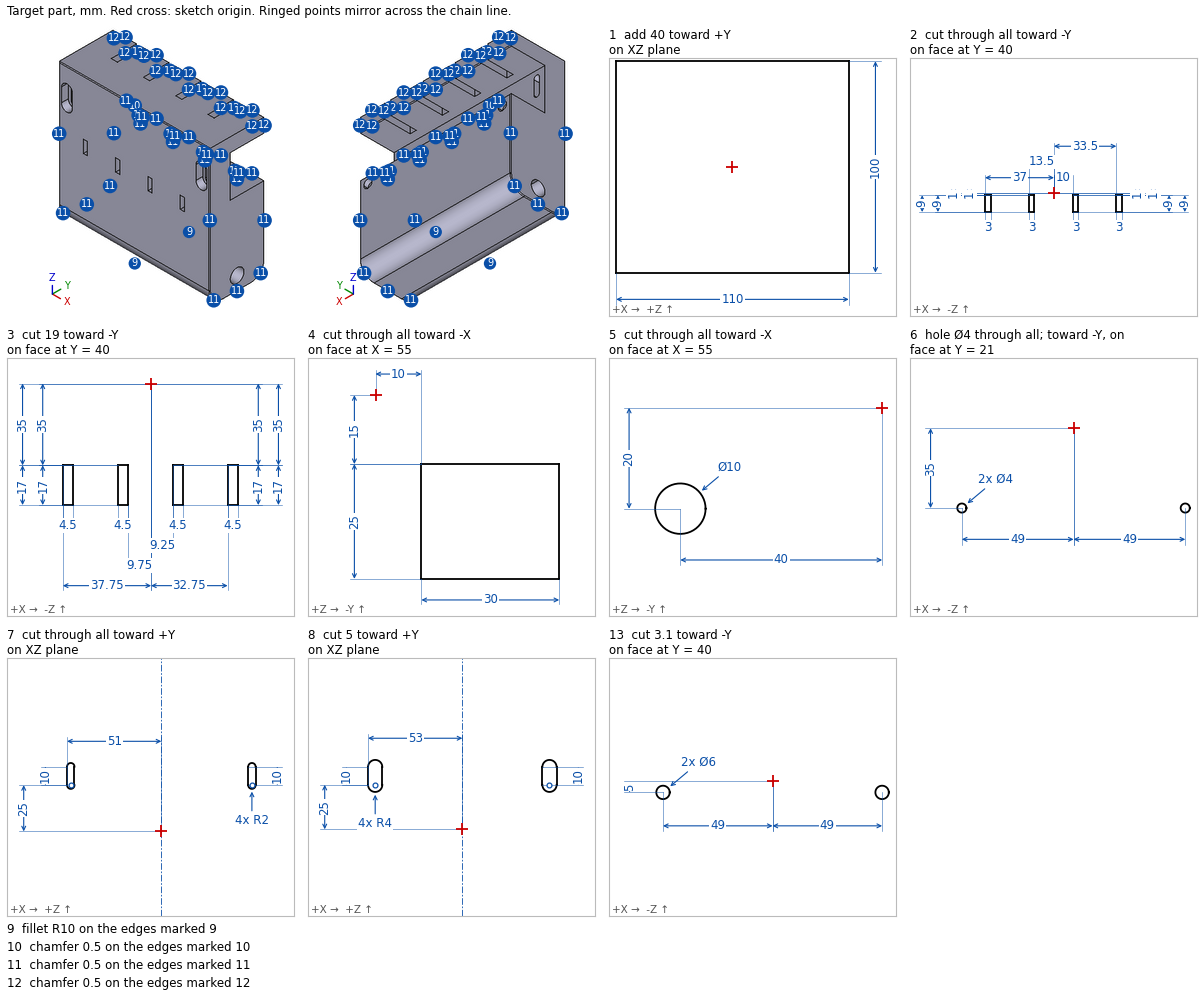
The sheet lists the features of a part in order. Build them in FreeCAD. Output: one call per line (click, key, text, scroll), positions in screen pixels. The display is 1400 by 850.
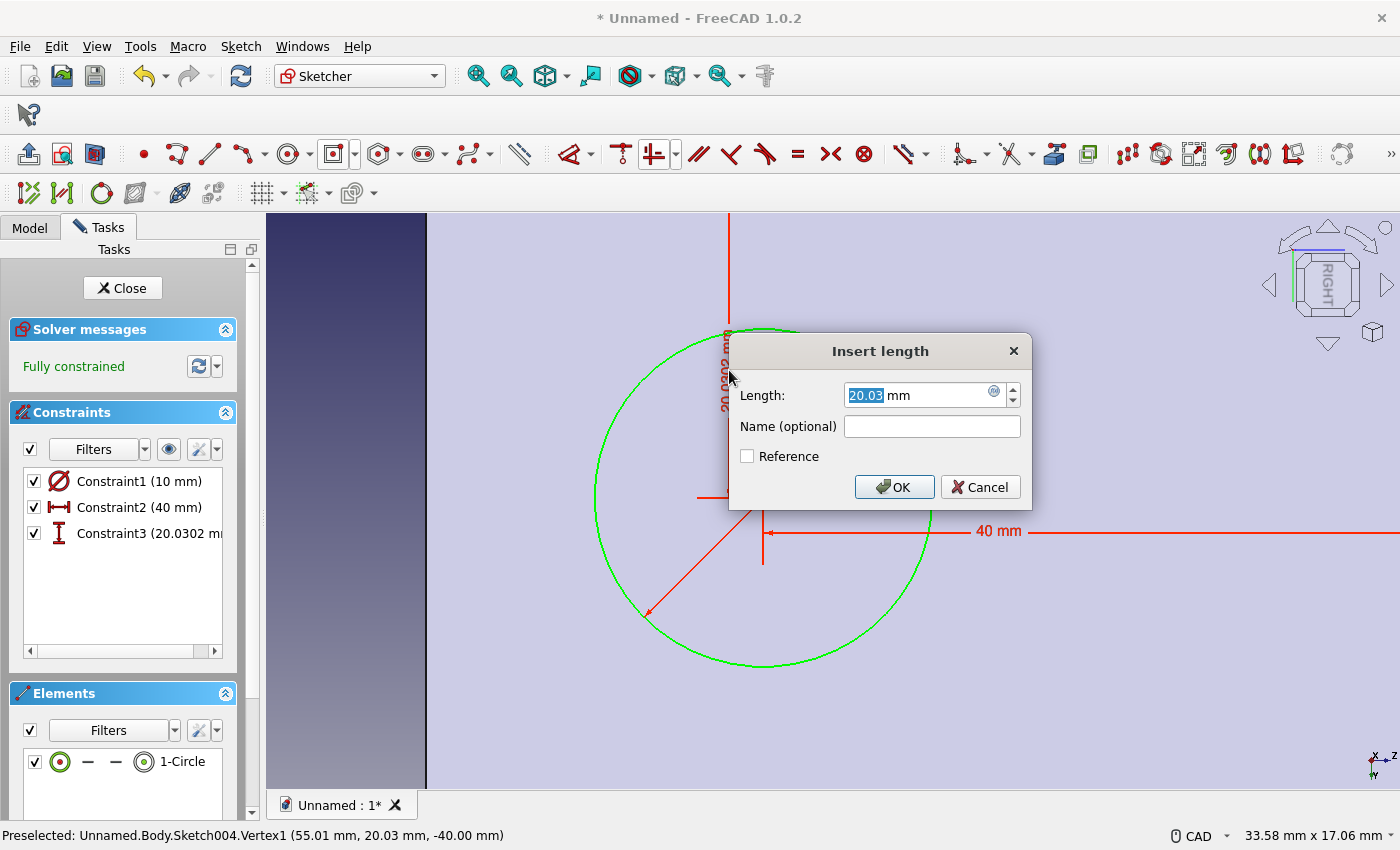
text(20)
key(Return)
key(Escape)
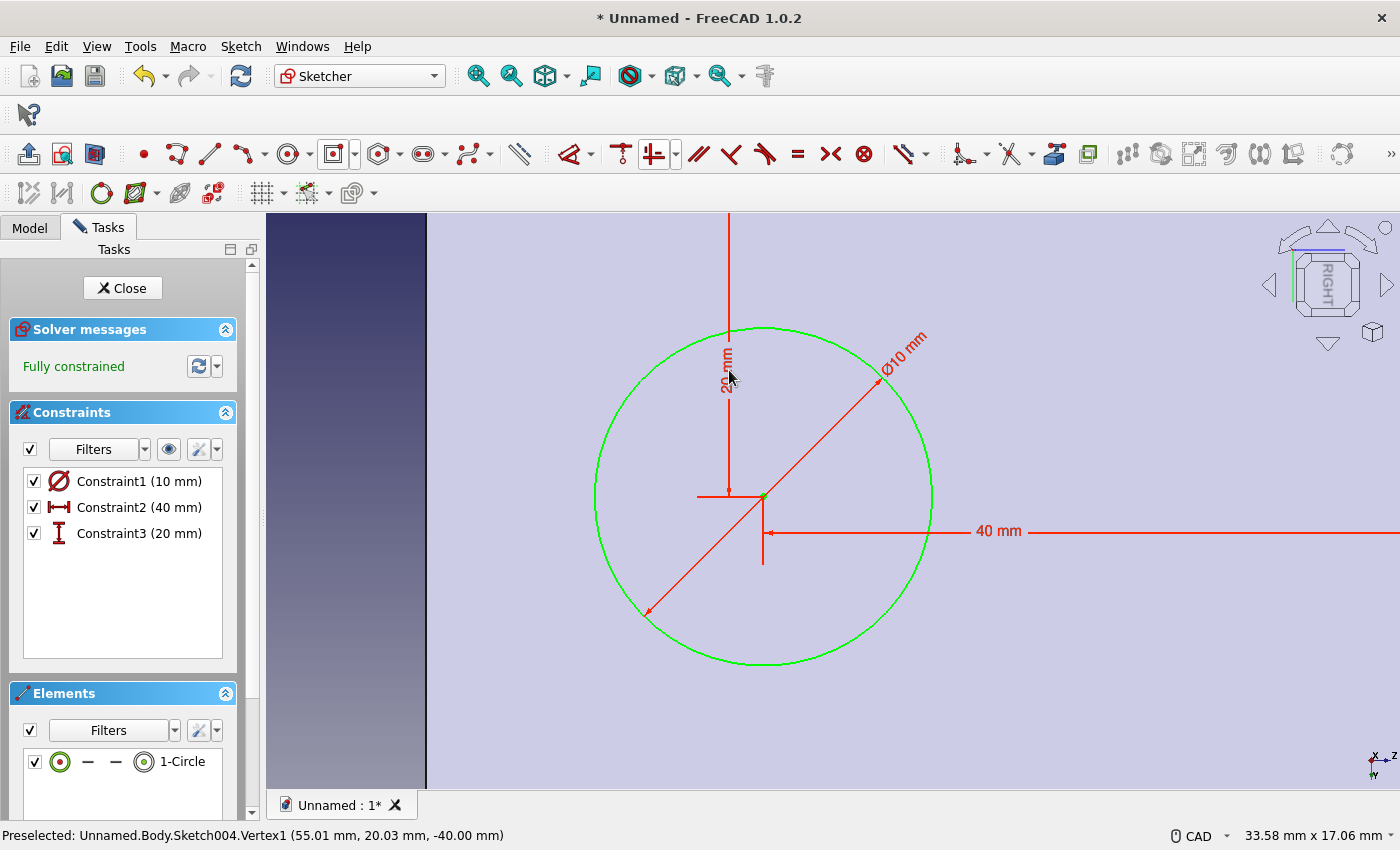
click(123, 288)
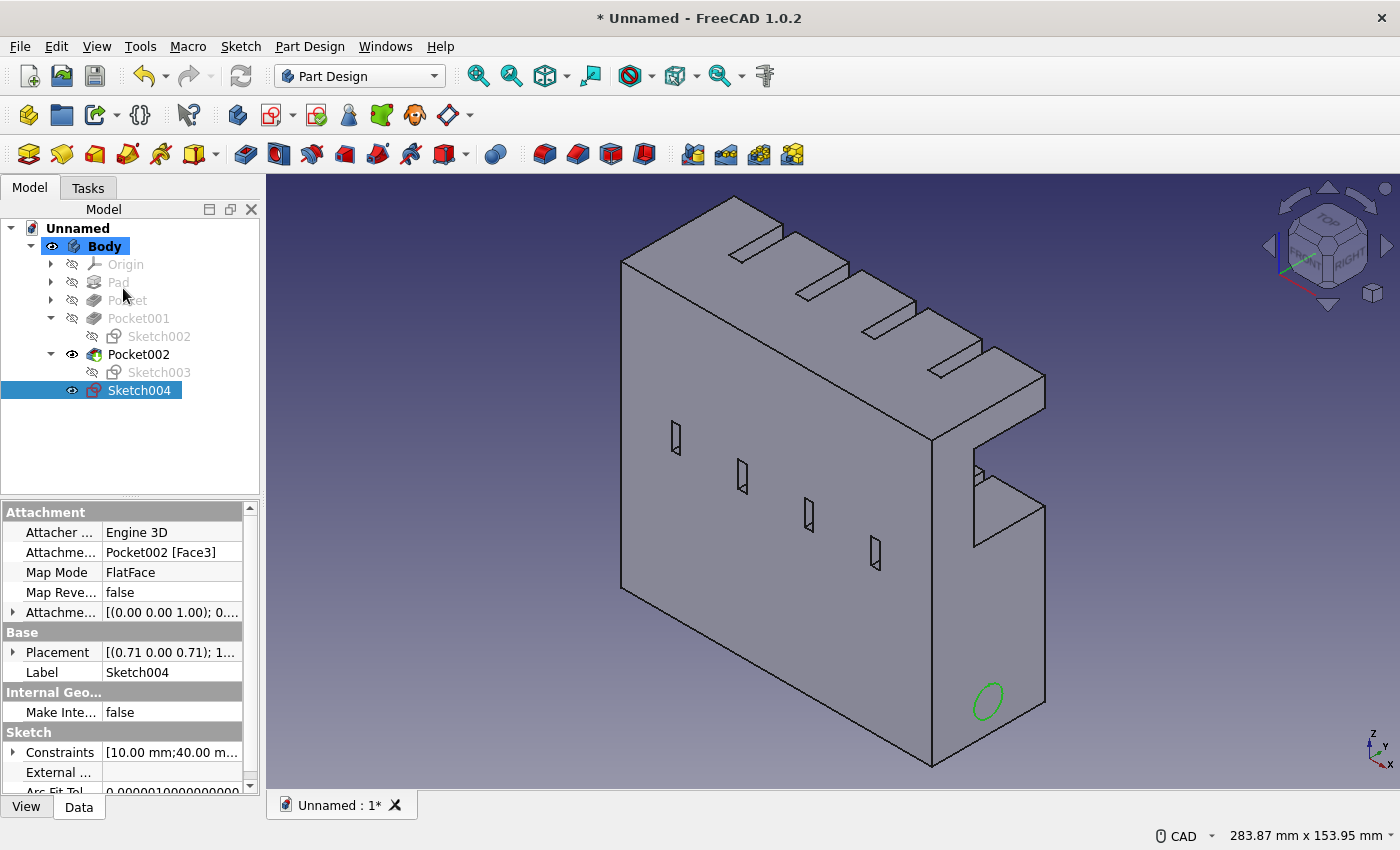
click(246, 154)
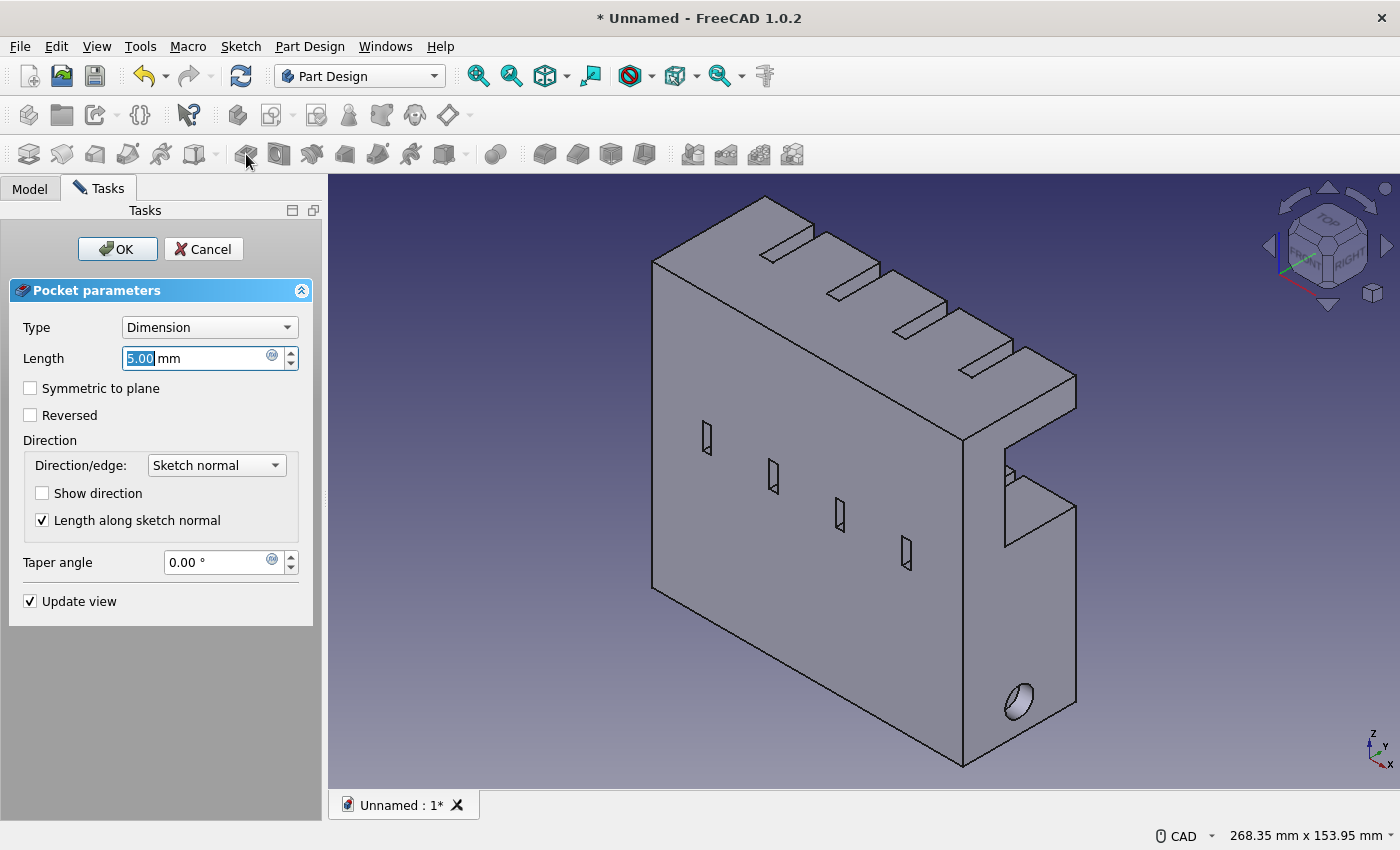
click(210, 328)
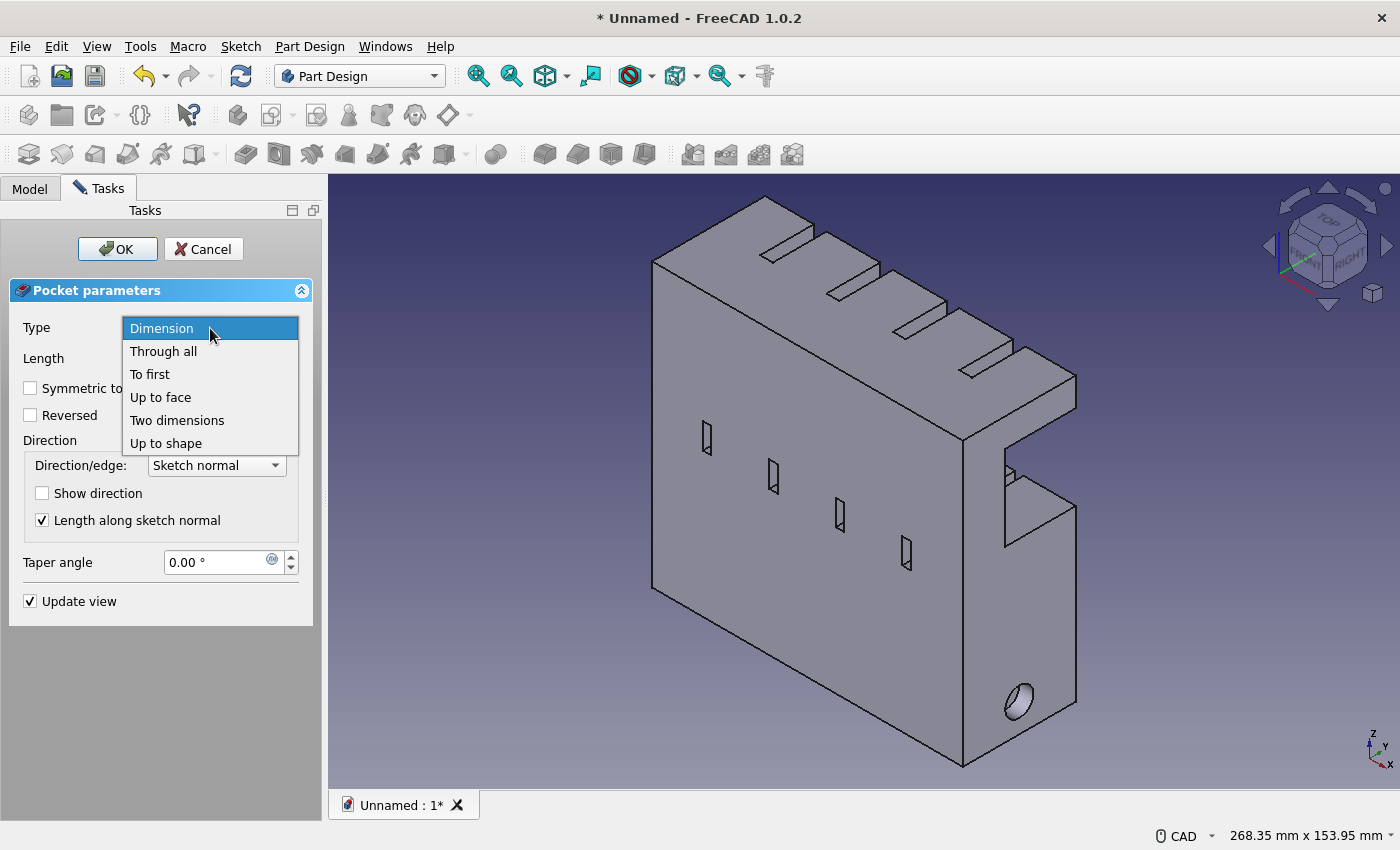
click(208, 352)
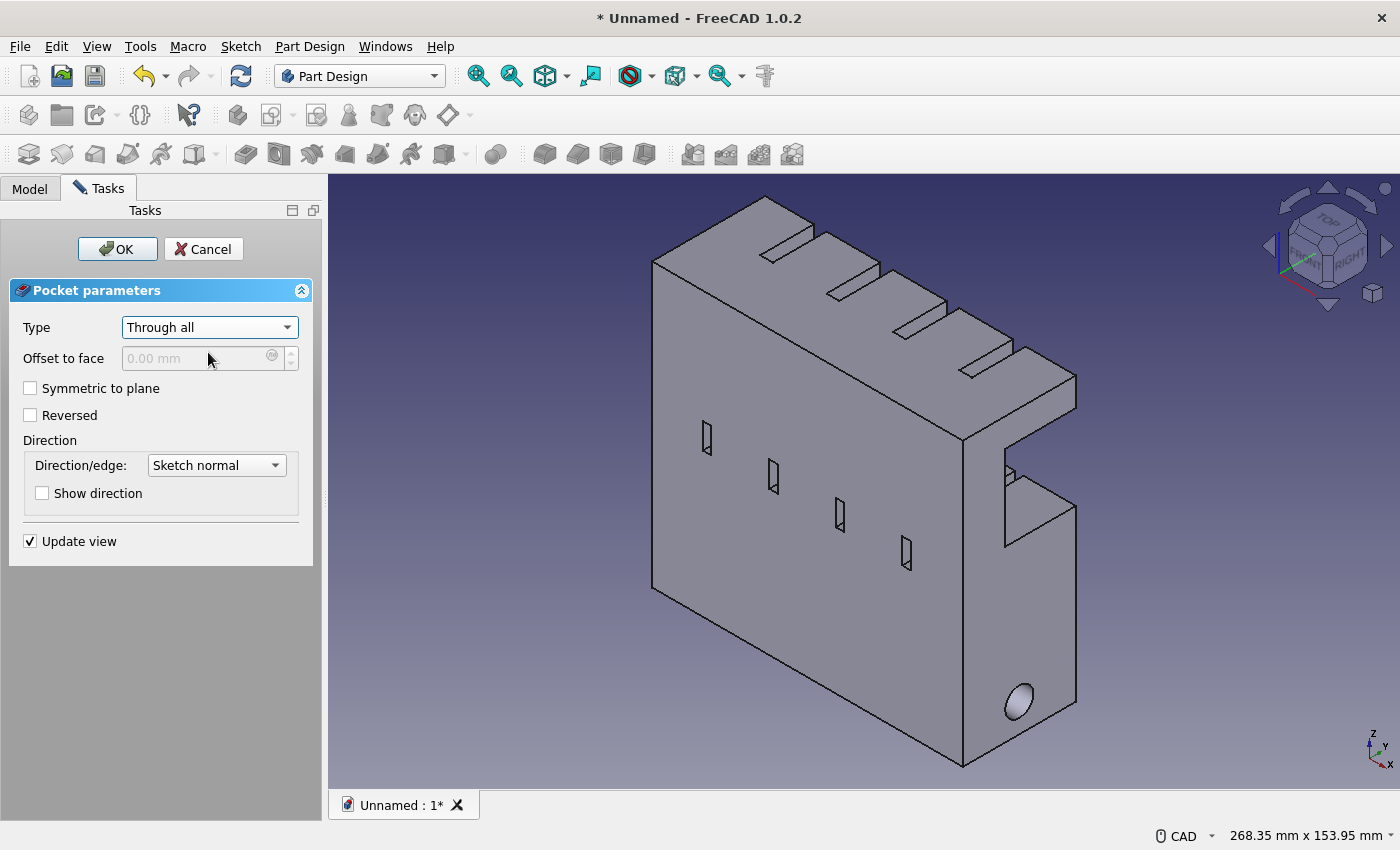
click(118, 249)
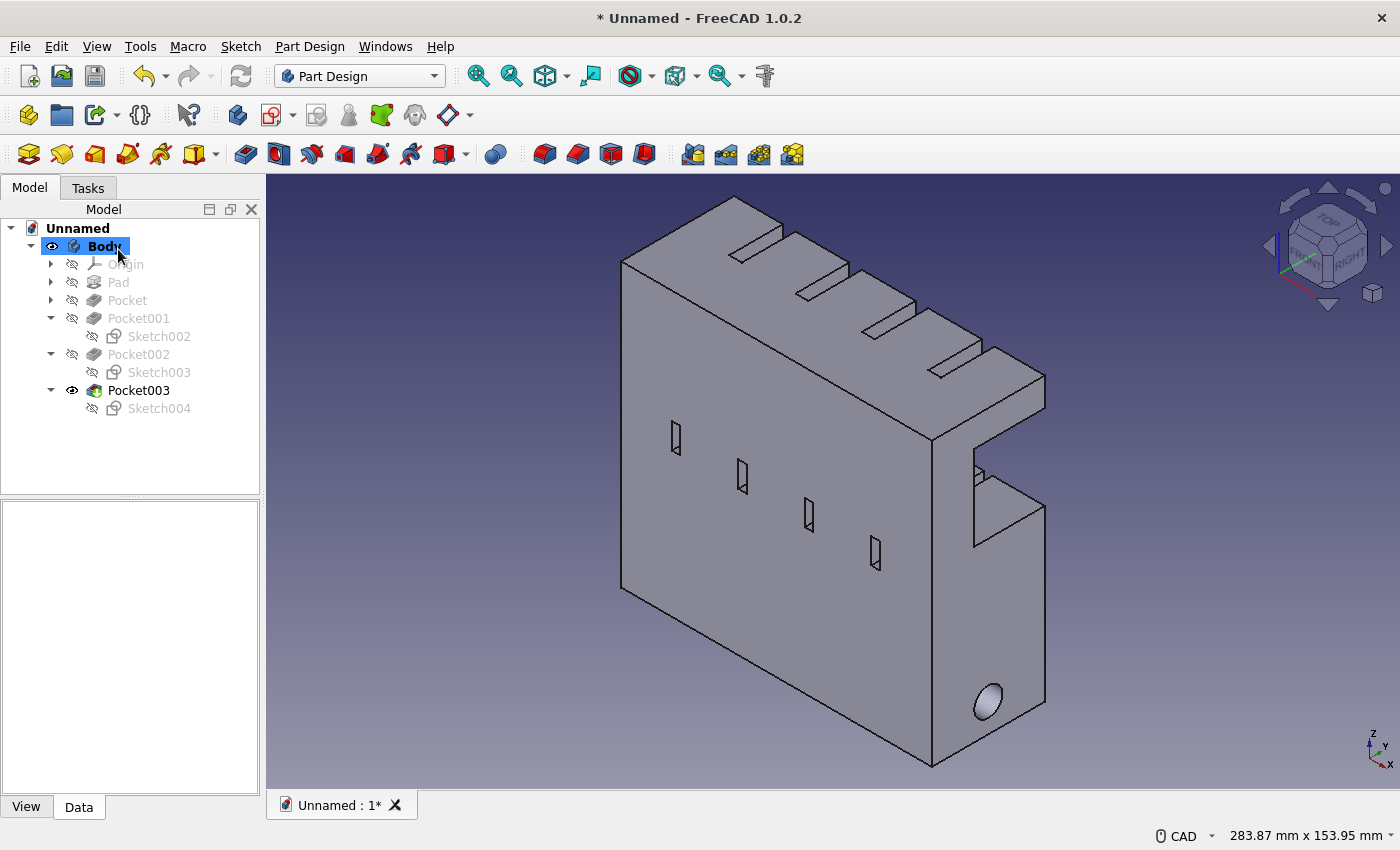
key(4)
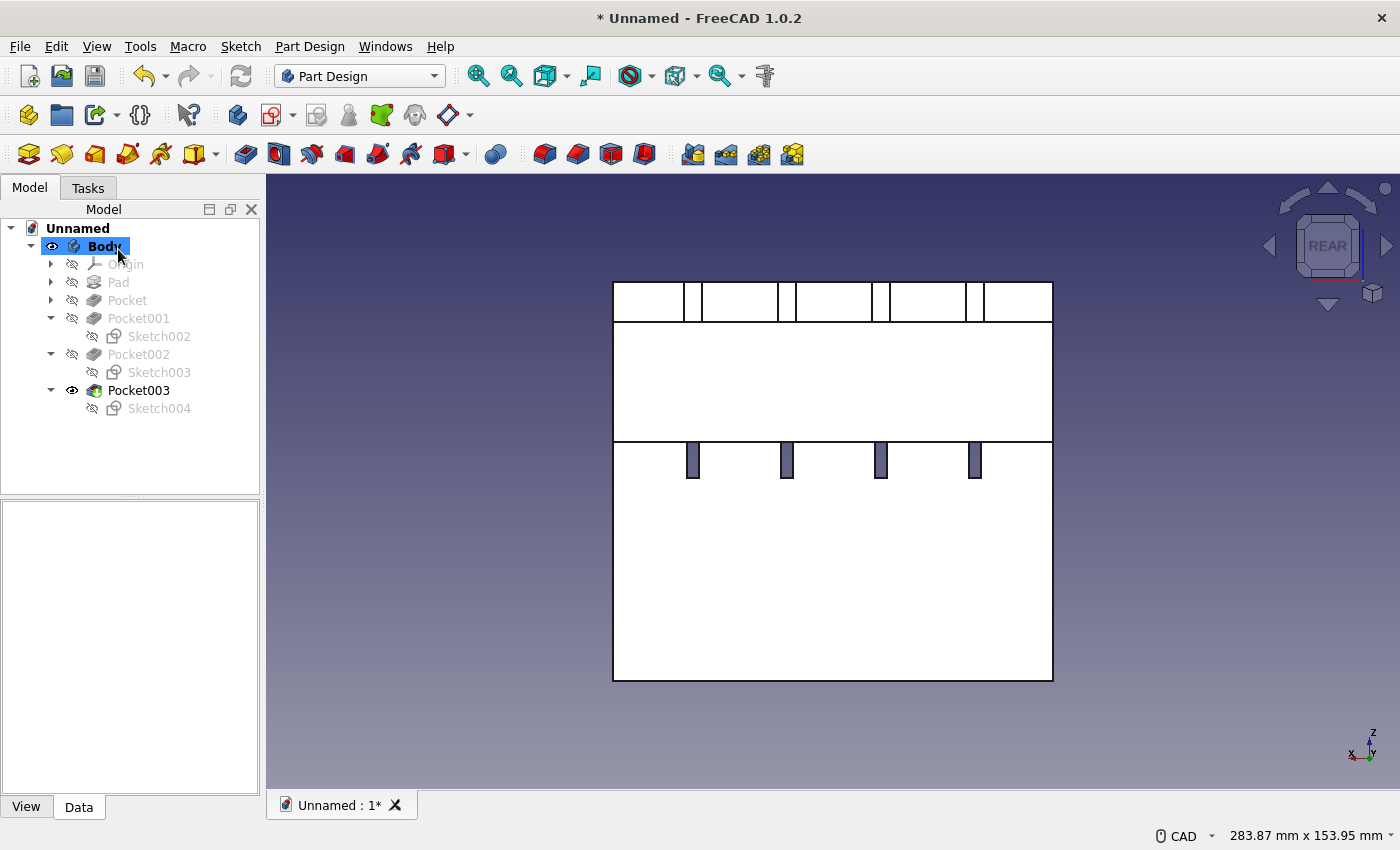
click(693, 295)